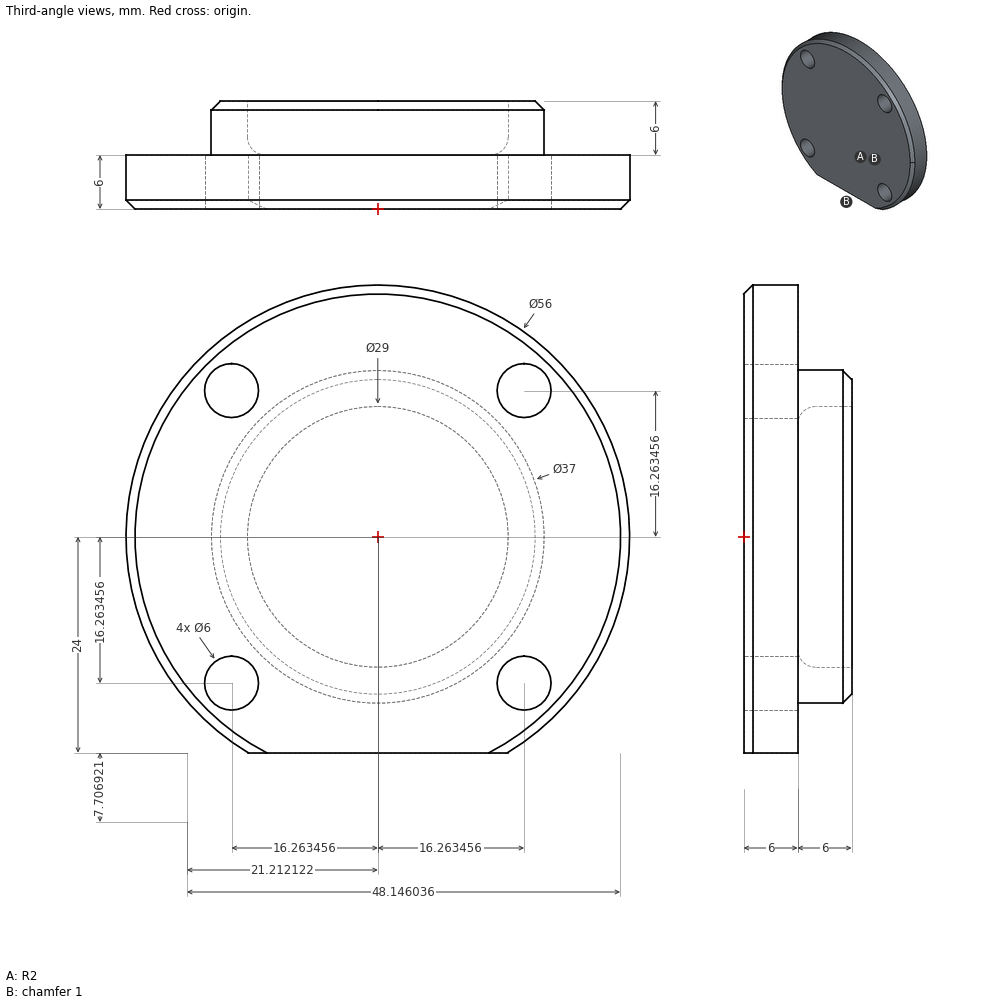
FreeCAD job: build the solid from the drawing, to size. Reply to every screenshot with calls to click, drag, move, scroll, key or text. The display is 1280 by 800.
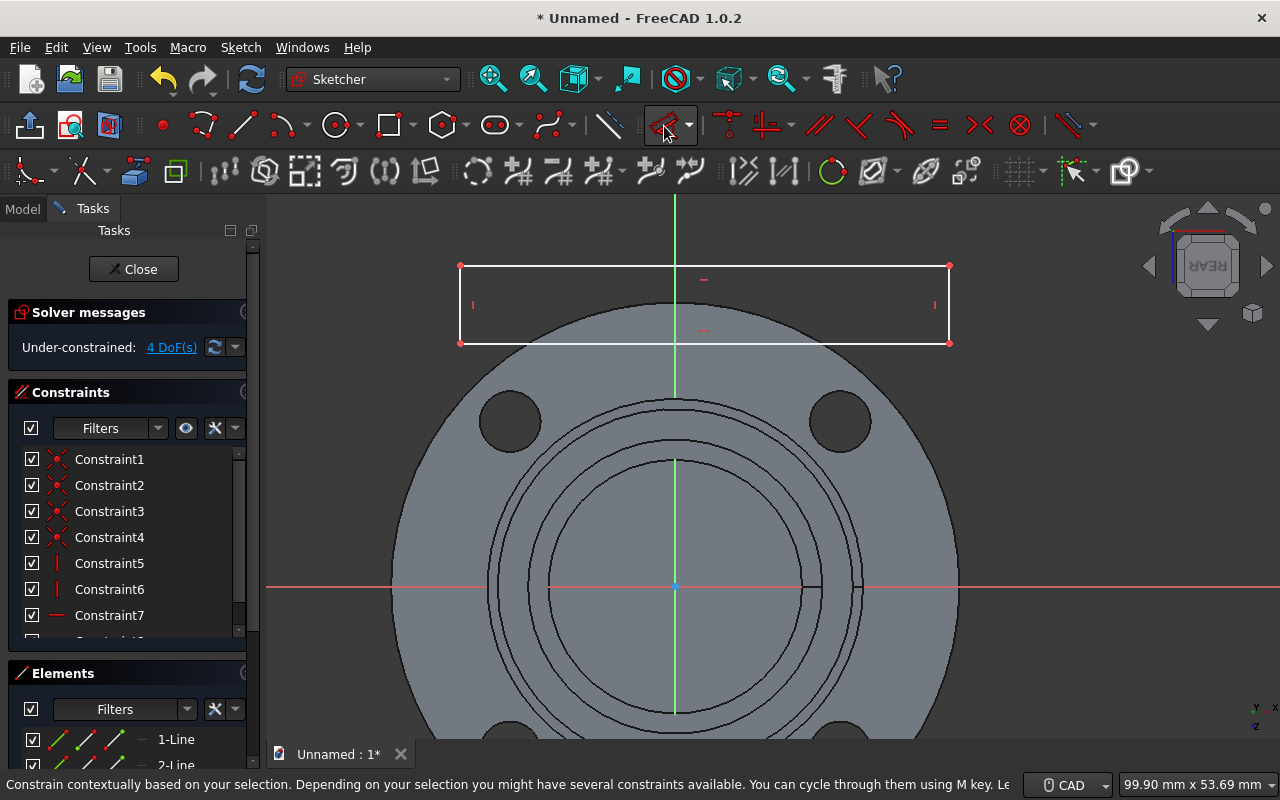
click(460, 344)
click(426, 465)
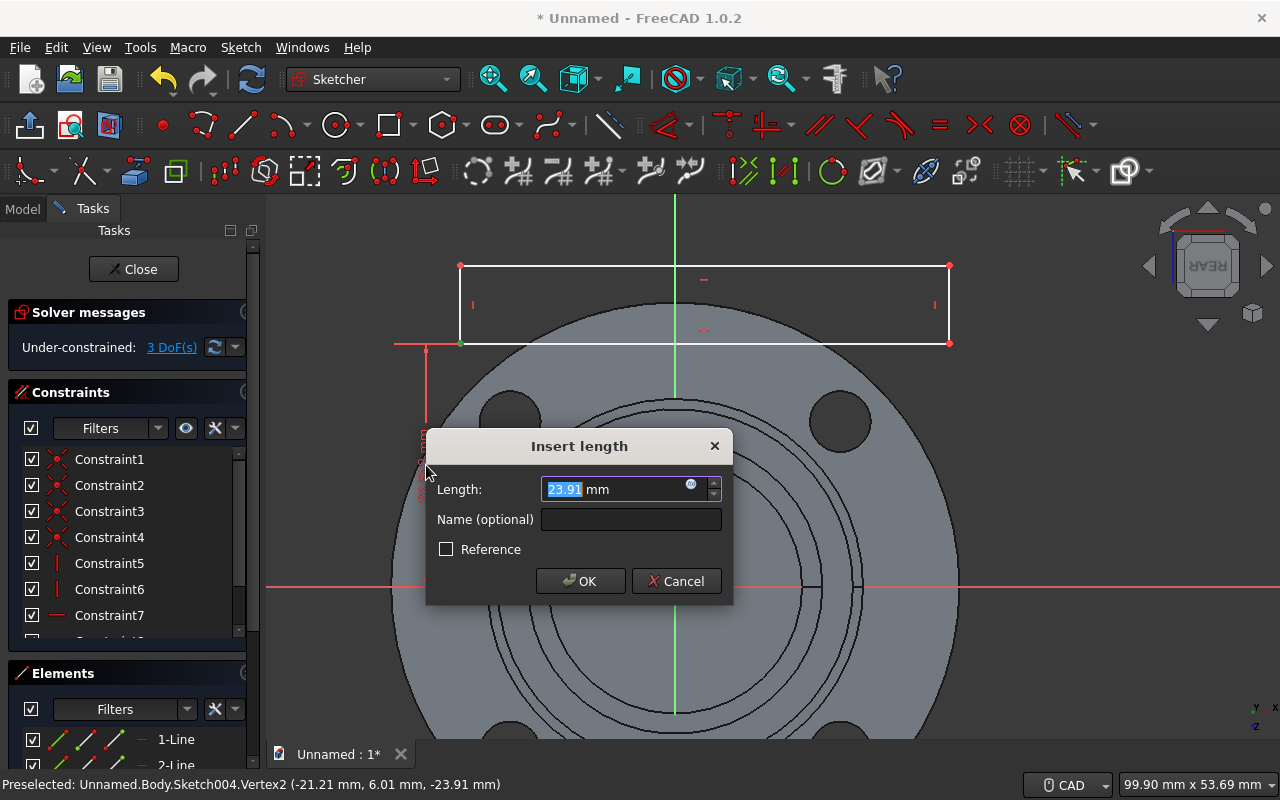
text(24)
key(Return)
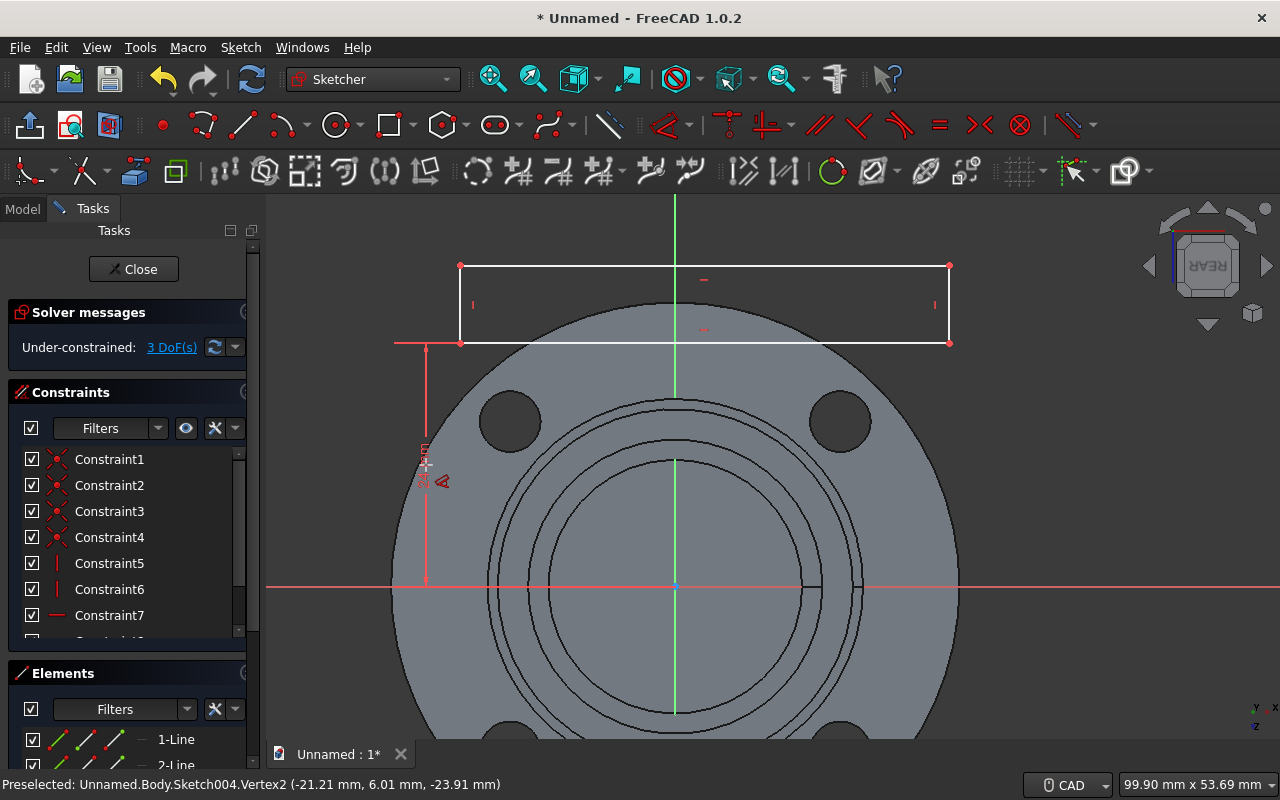
click(460, 289)
click(426, 305)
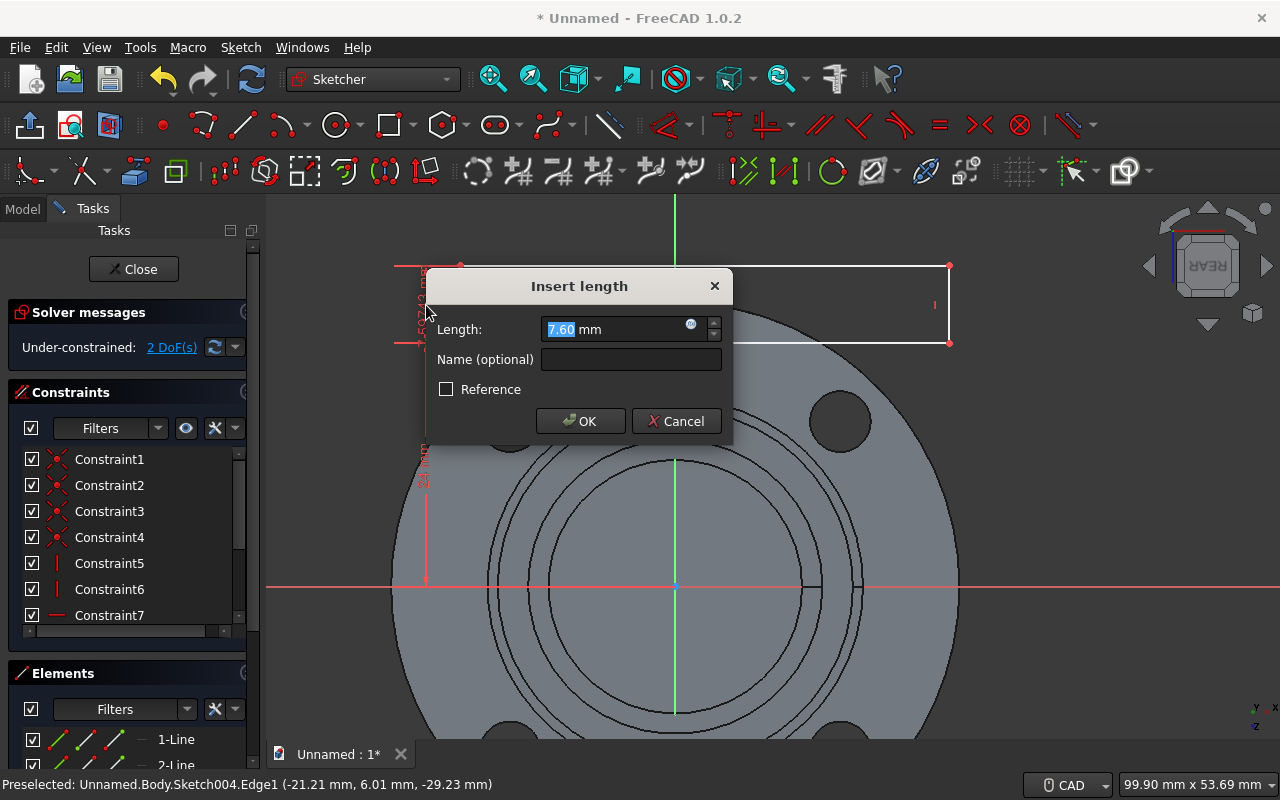
text(7.706921)
key(Return)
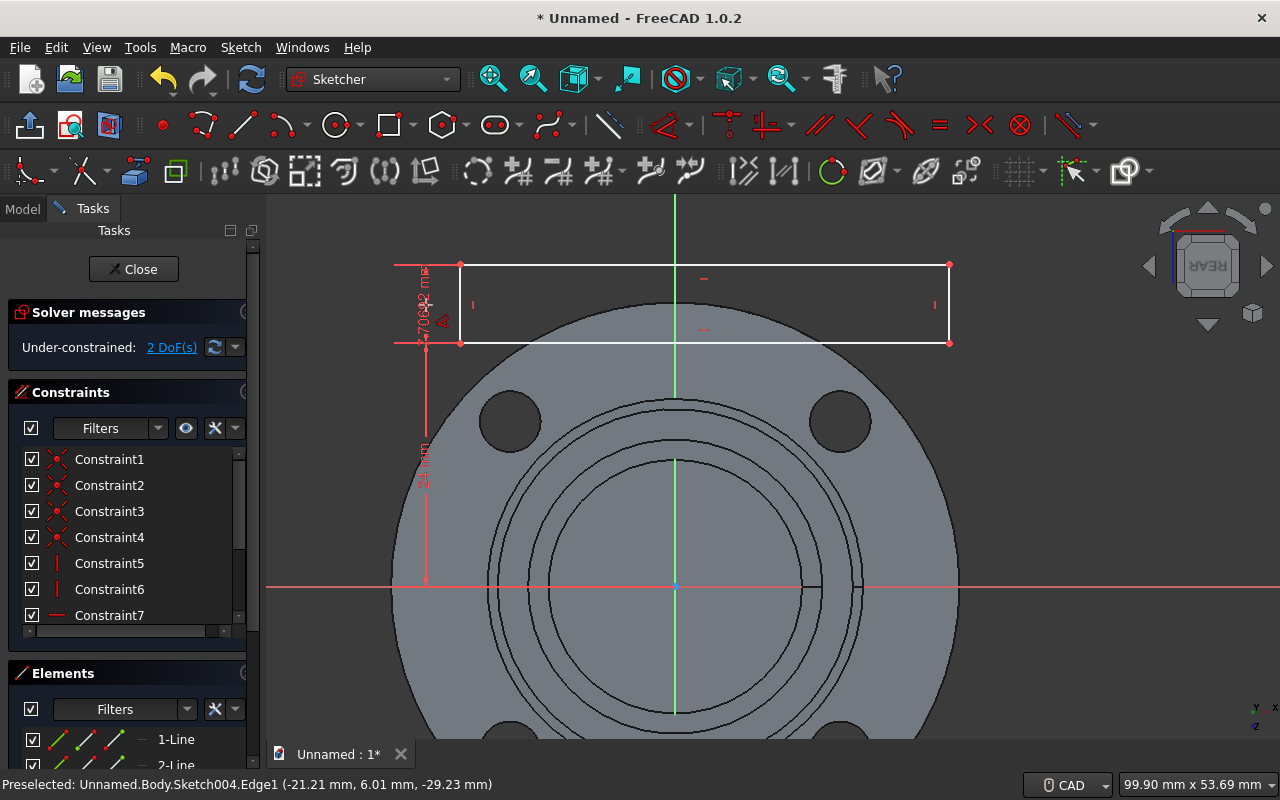
click(607, 343)
click(705, 309)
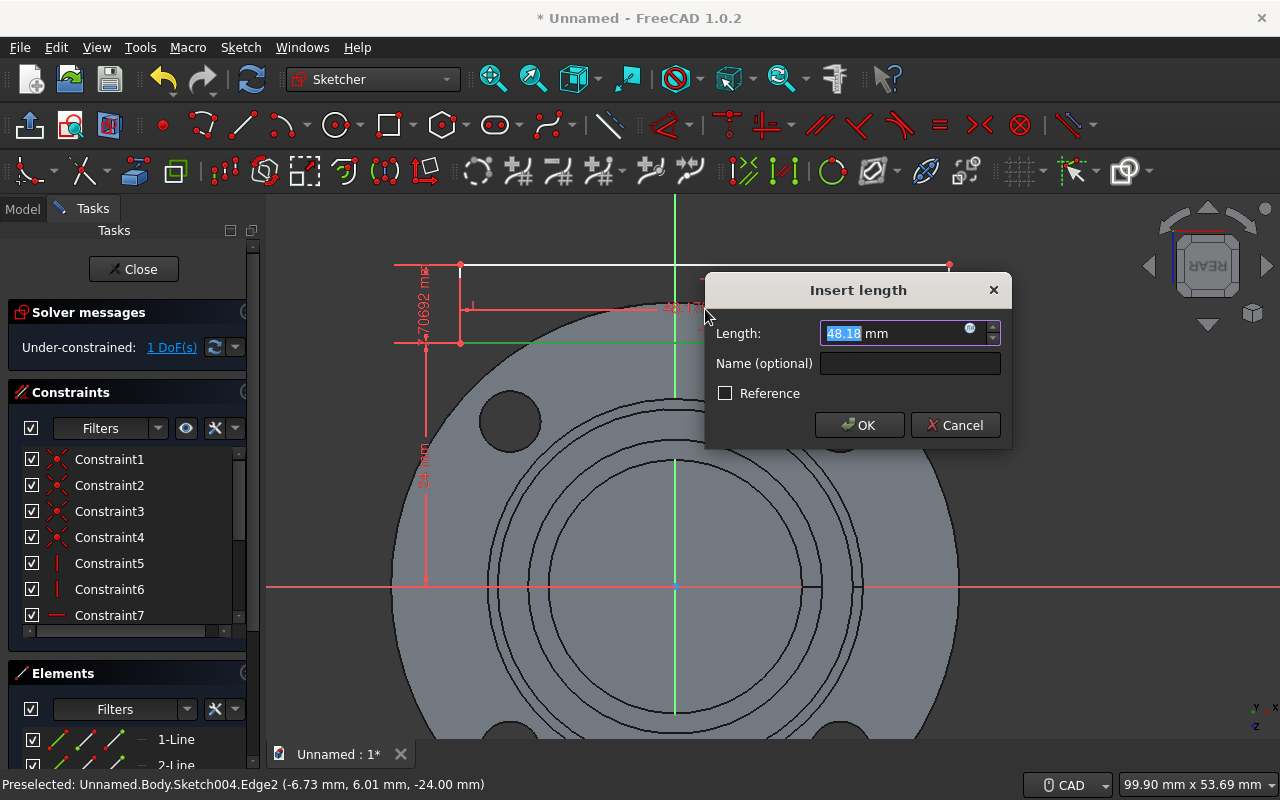
text(48.146036)
key(Return)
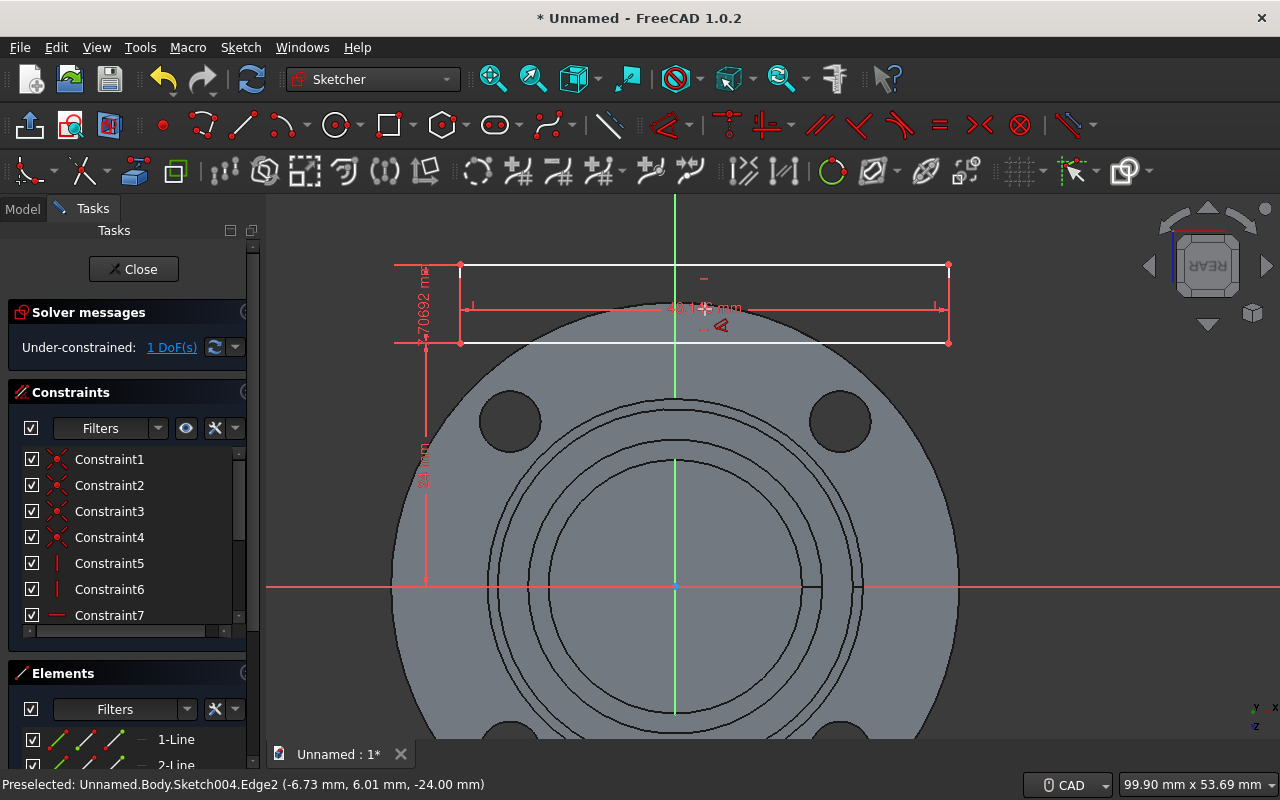
click(460, 265)
click(568, 621)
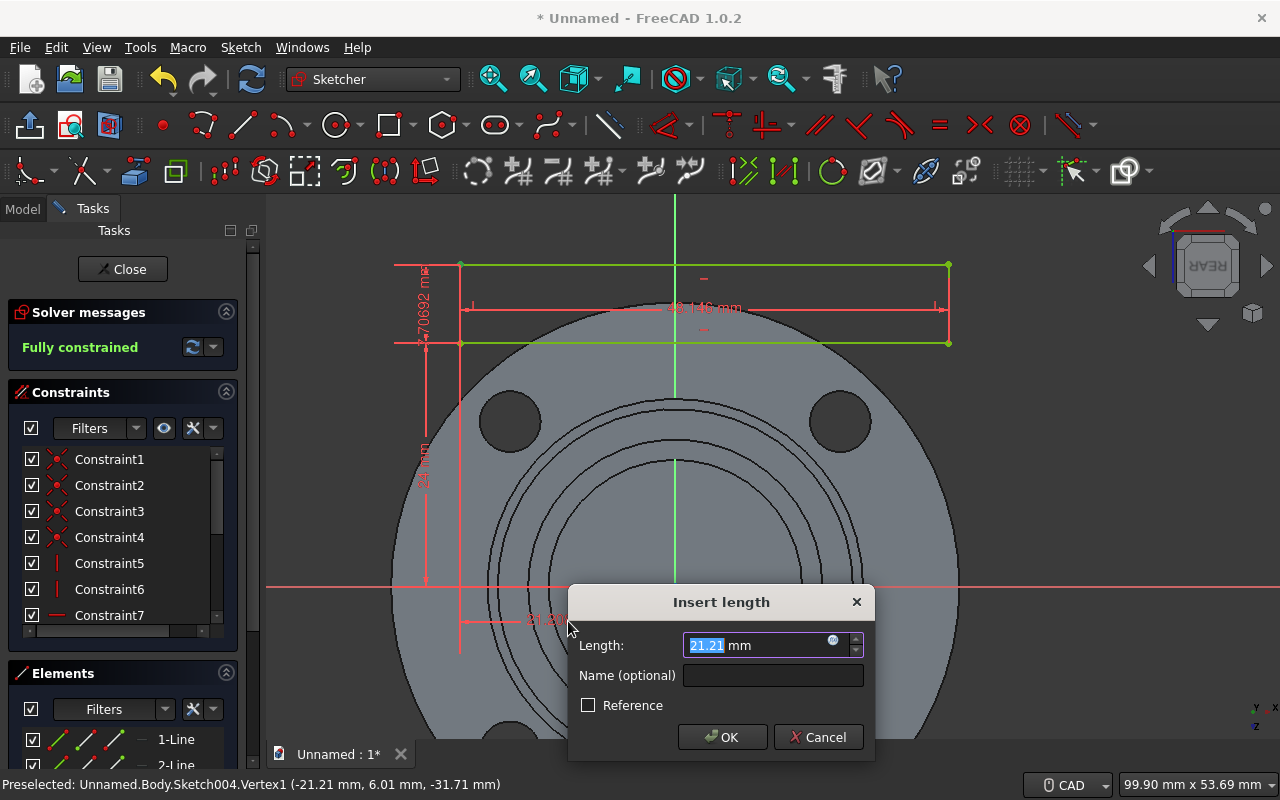
text(21.212122)
key(Return)
key(Escape)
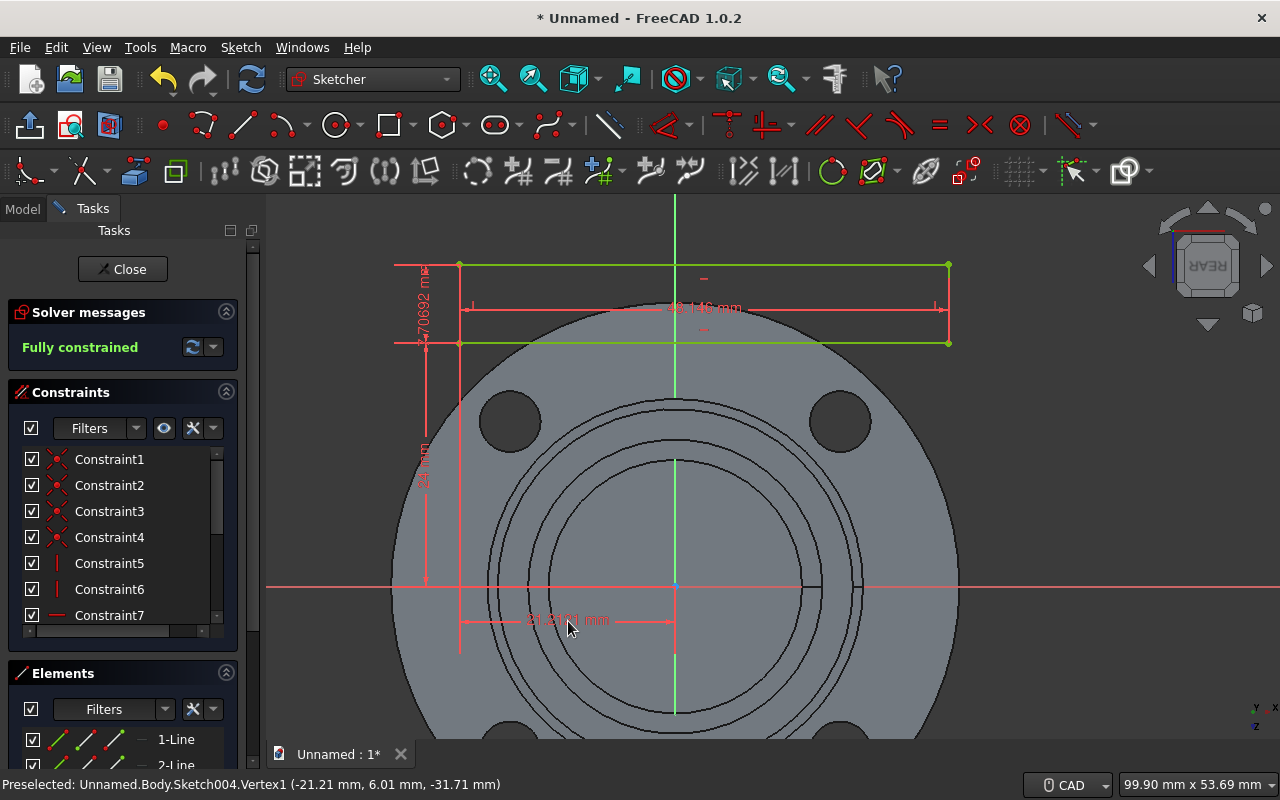
click(123, 269)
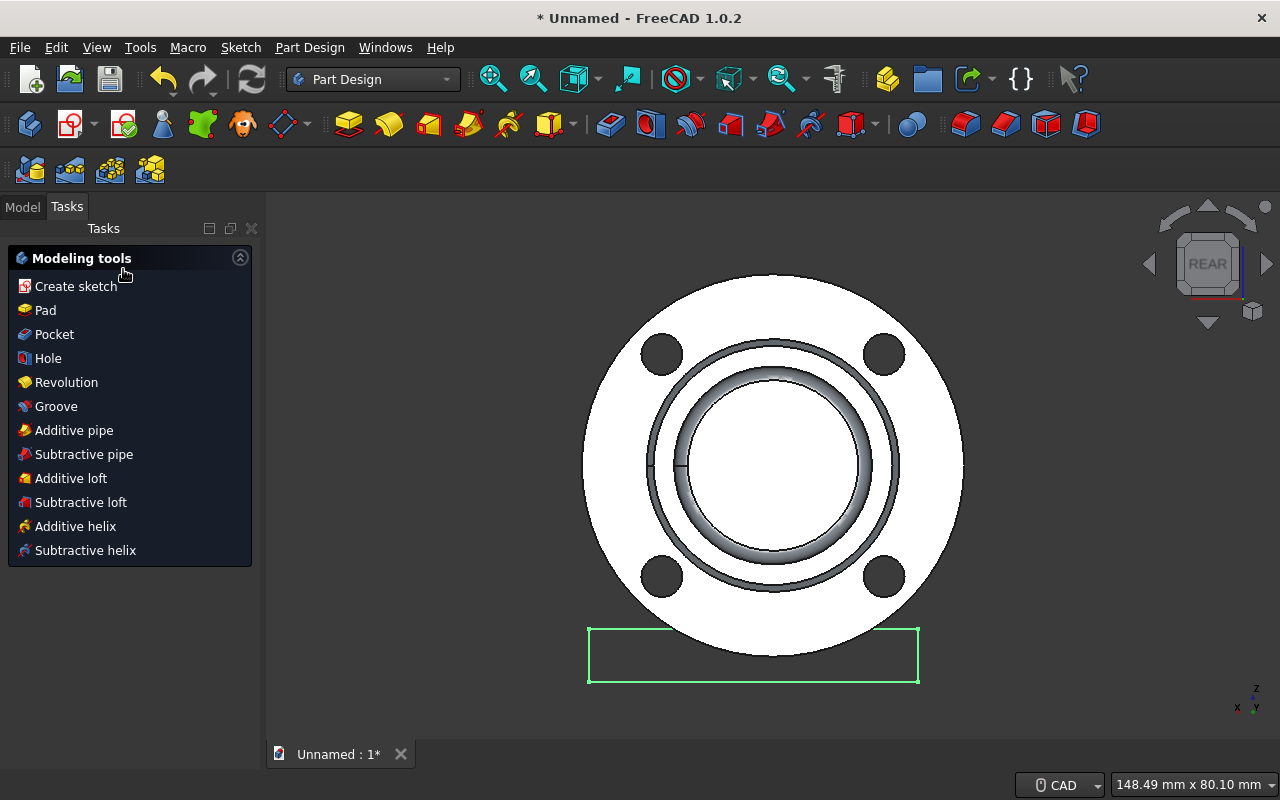
click(612, 124)